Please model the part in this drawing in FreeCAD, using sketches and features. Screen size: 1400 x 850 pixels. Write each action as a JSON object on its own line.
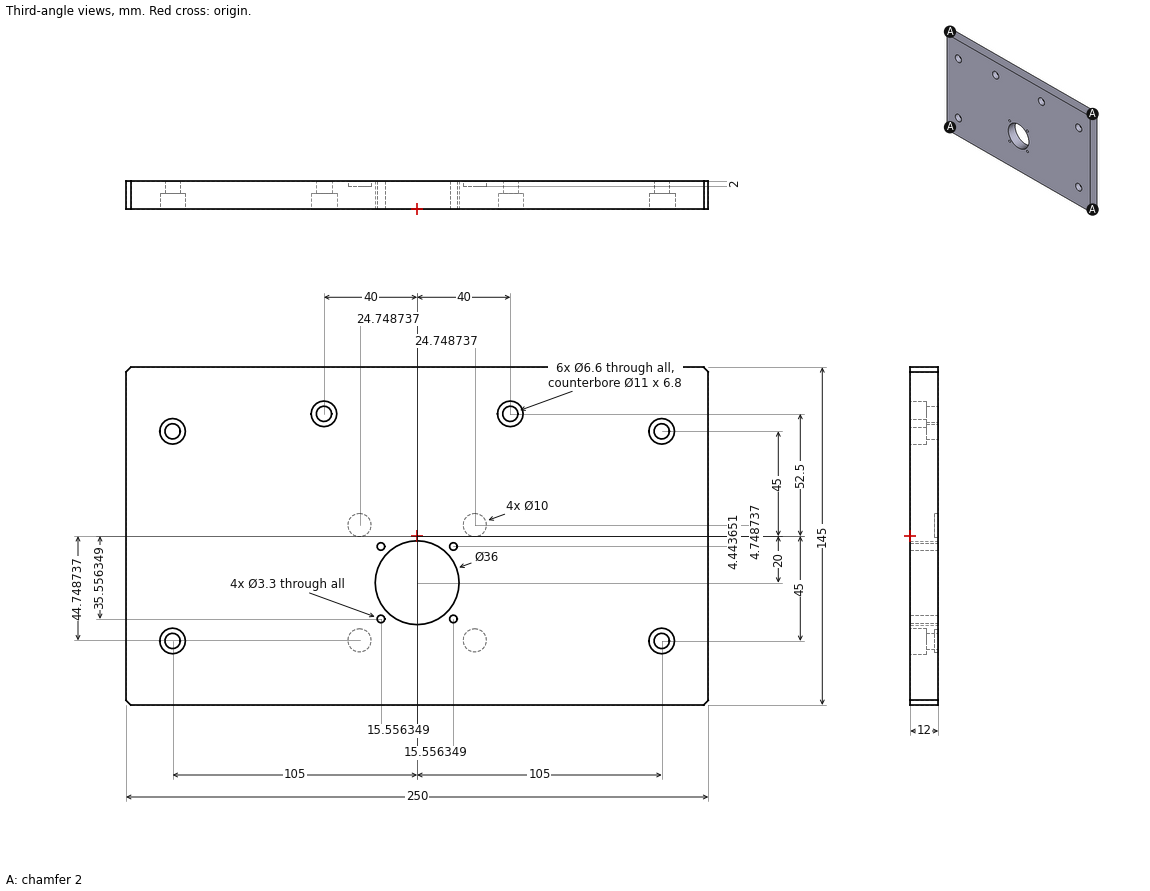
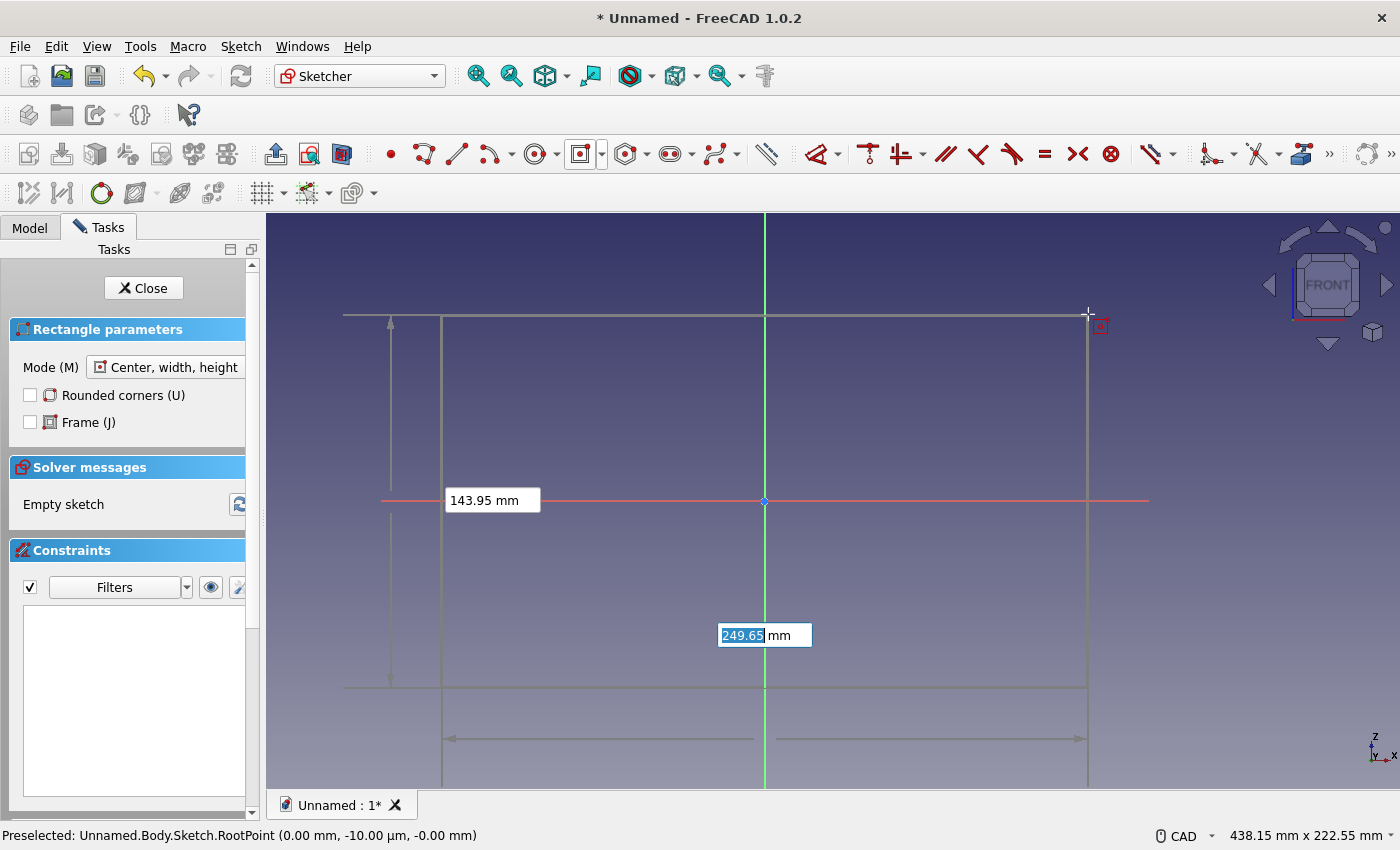
{"action": "type", "text": "250"}
{"action": "key", "text": "Tab"}
{"action": "type", "text": "145"}
{"action": "key", "text": "Return"}
{"action": "key", "text": "Escape"}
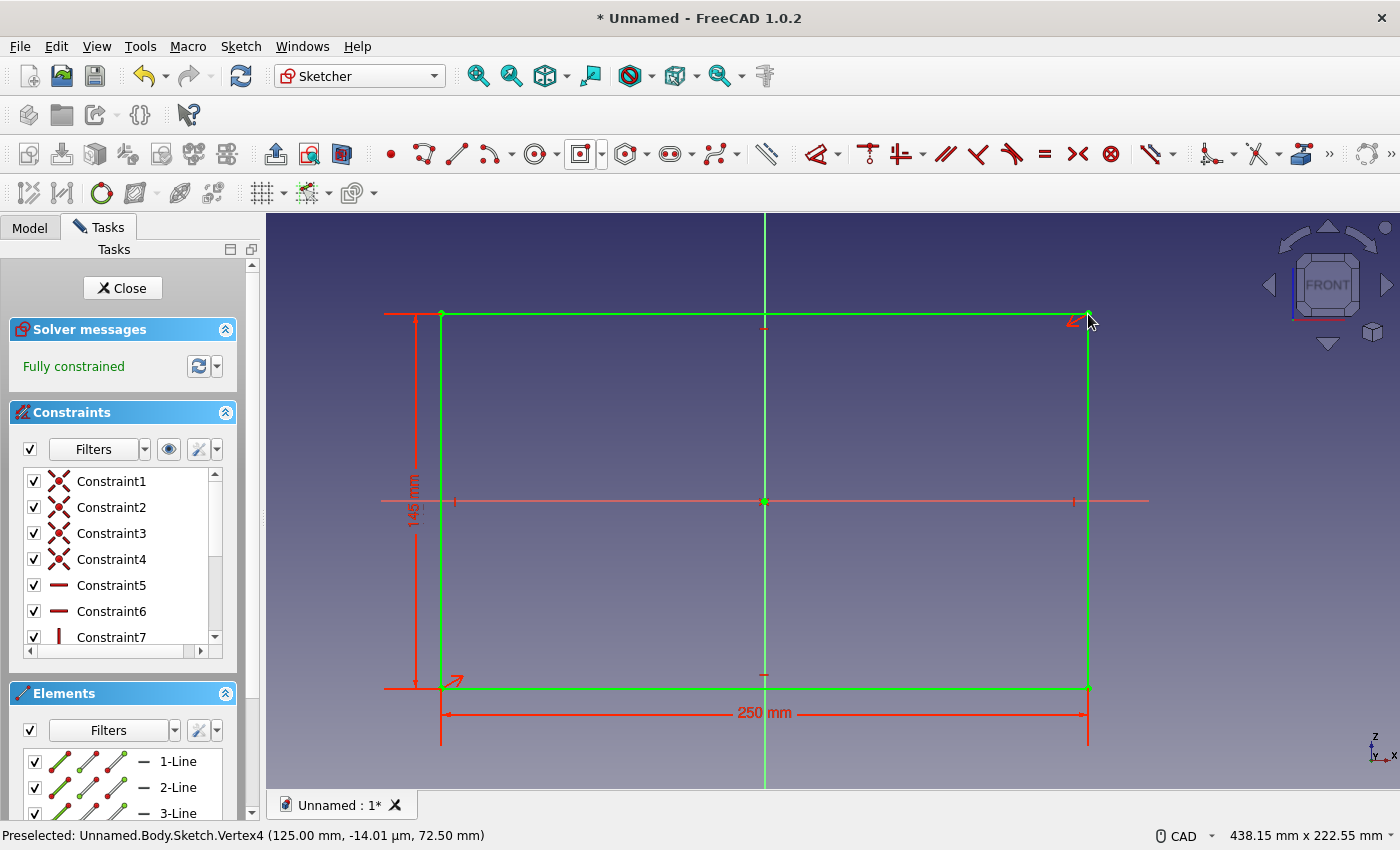
{"action": "left_click", "coordinate": [123, 288]}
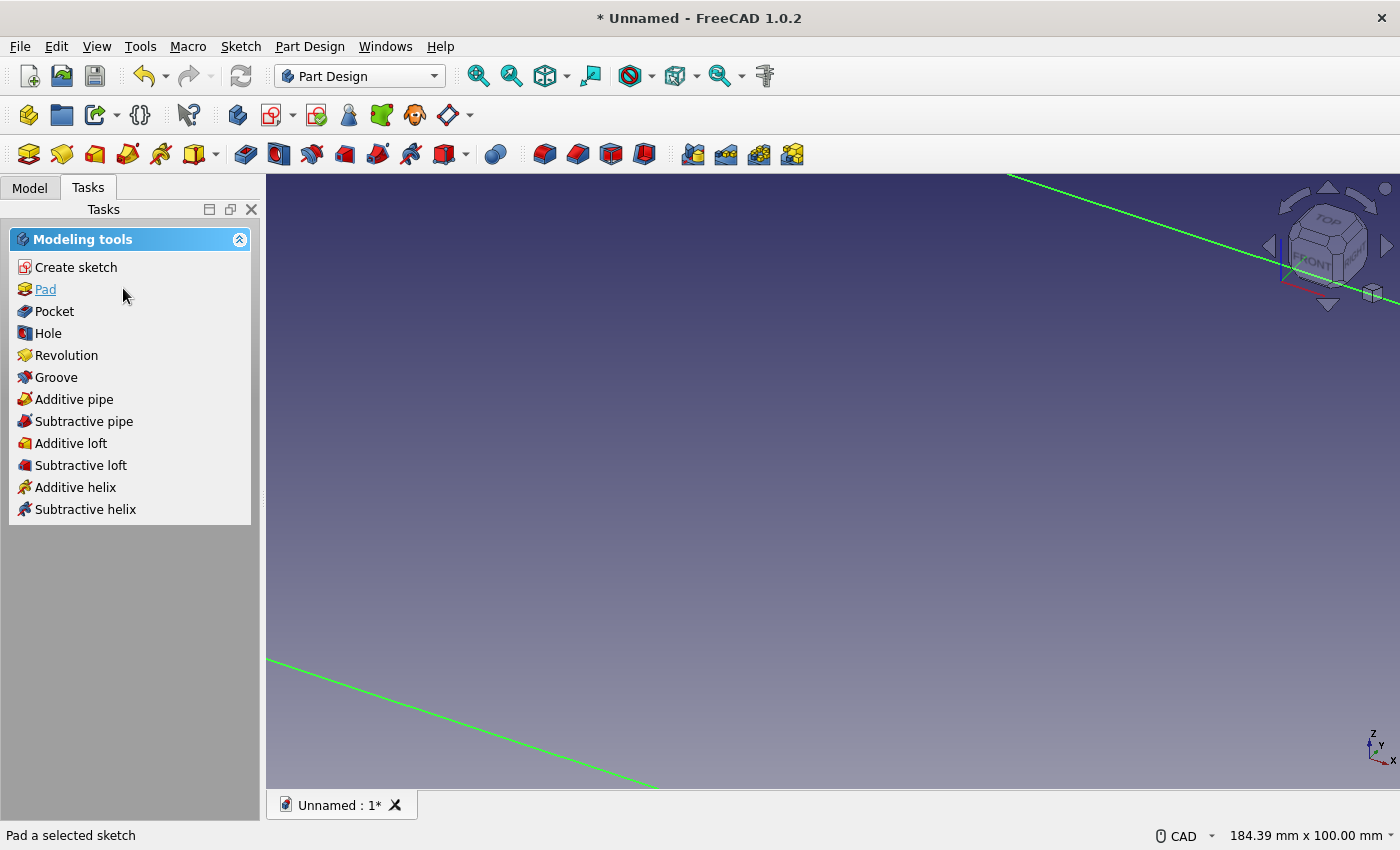
{"action": "left_click", "coordinate": [29, 154]}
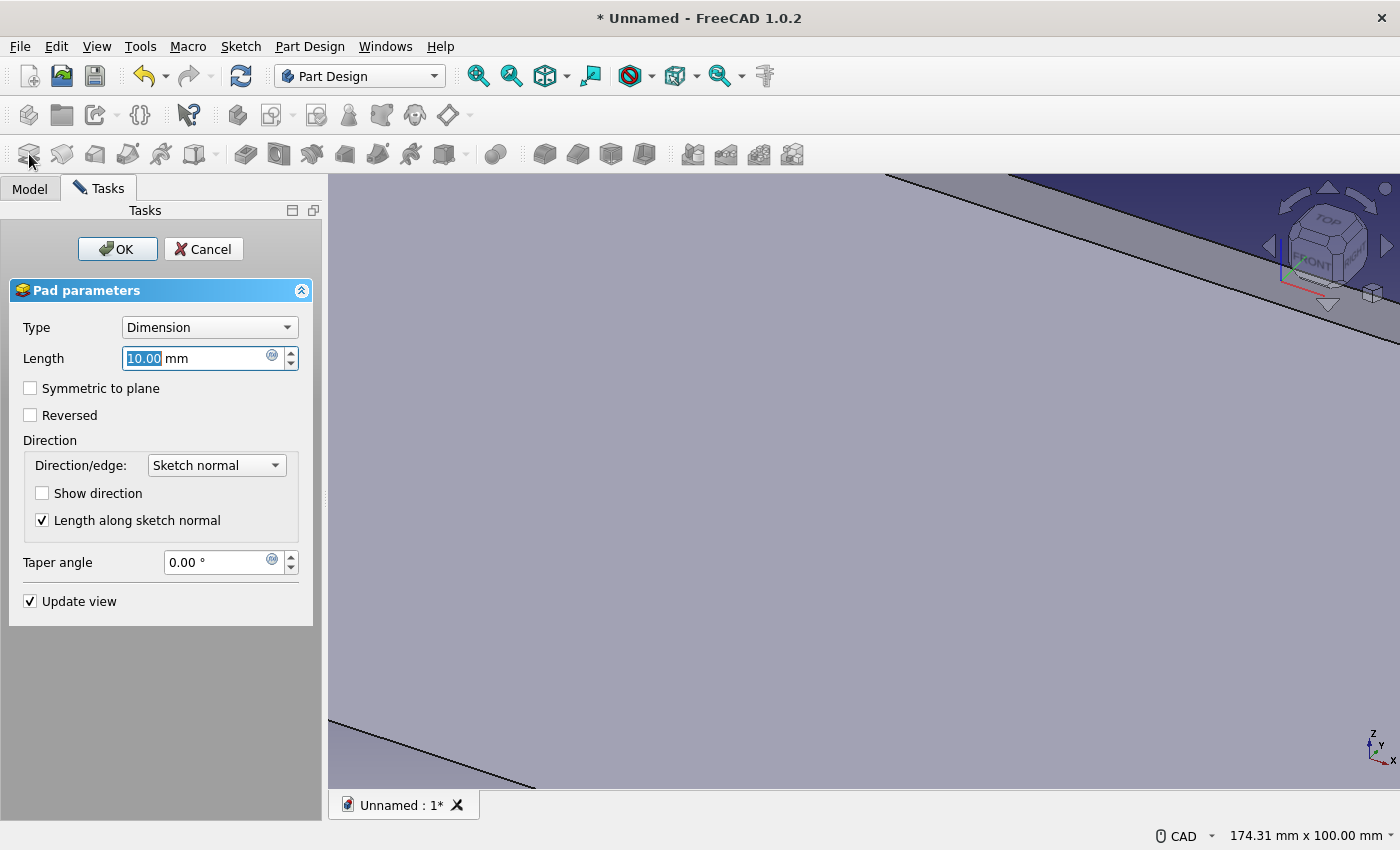
{"action": "type", "text": "12"}
{"action": "key", "text": "Tab"}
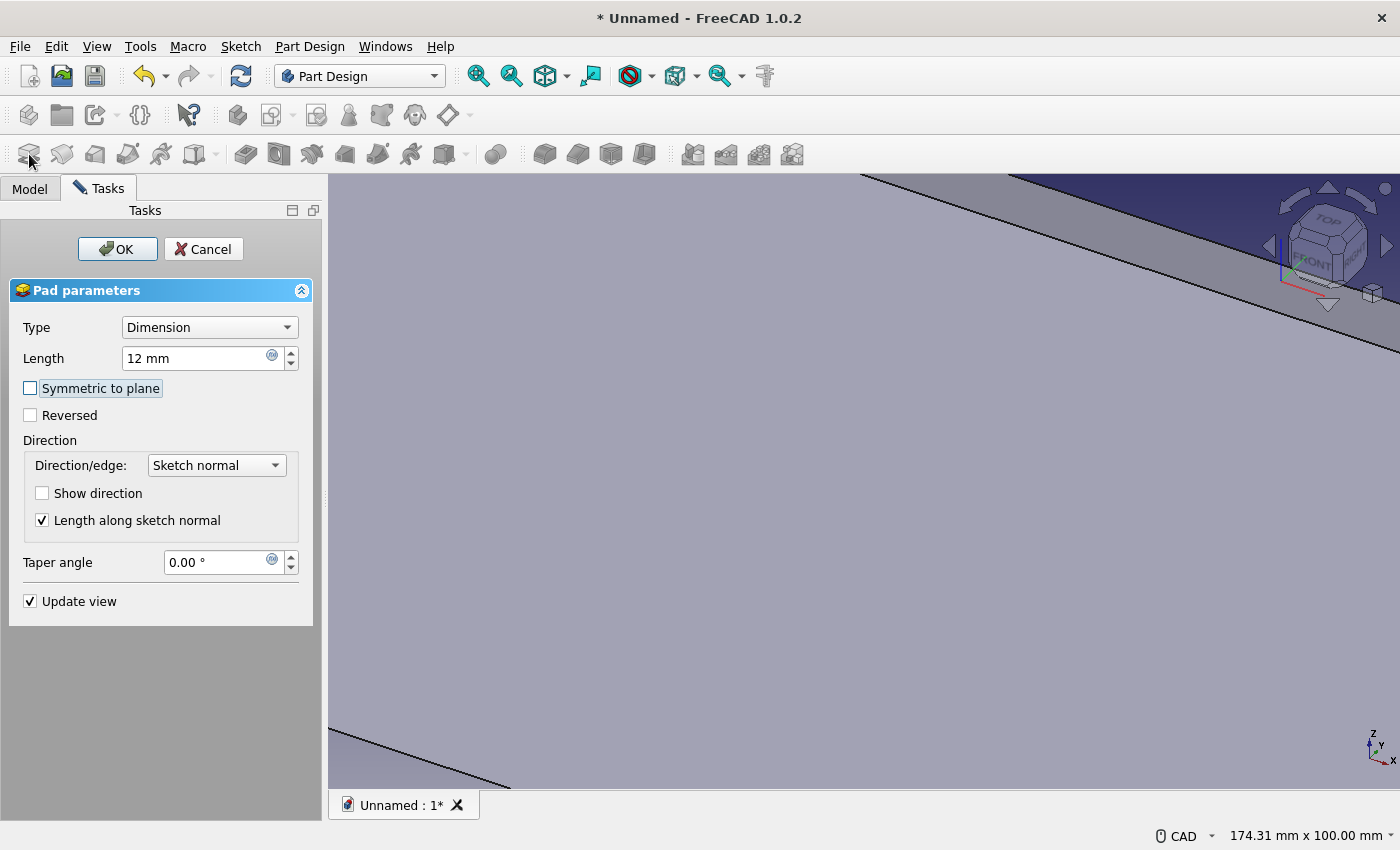
{"action": "left_click", "coordinate": [31, 415]}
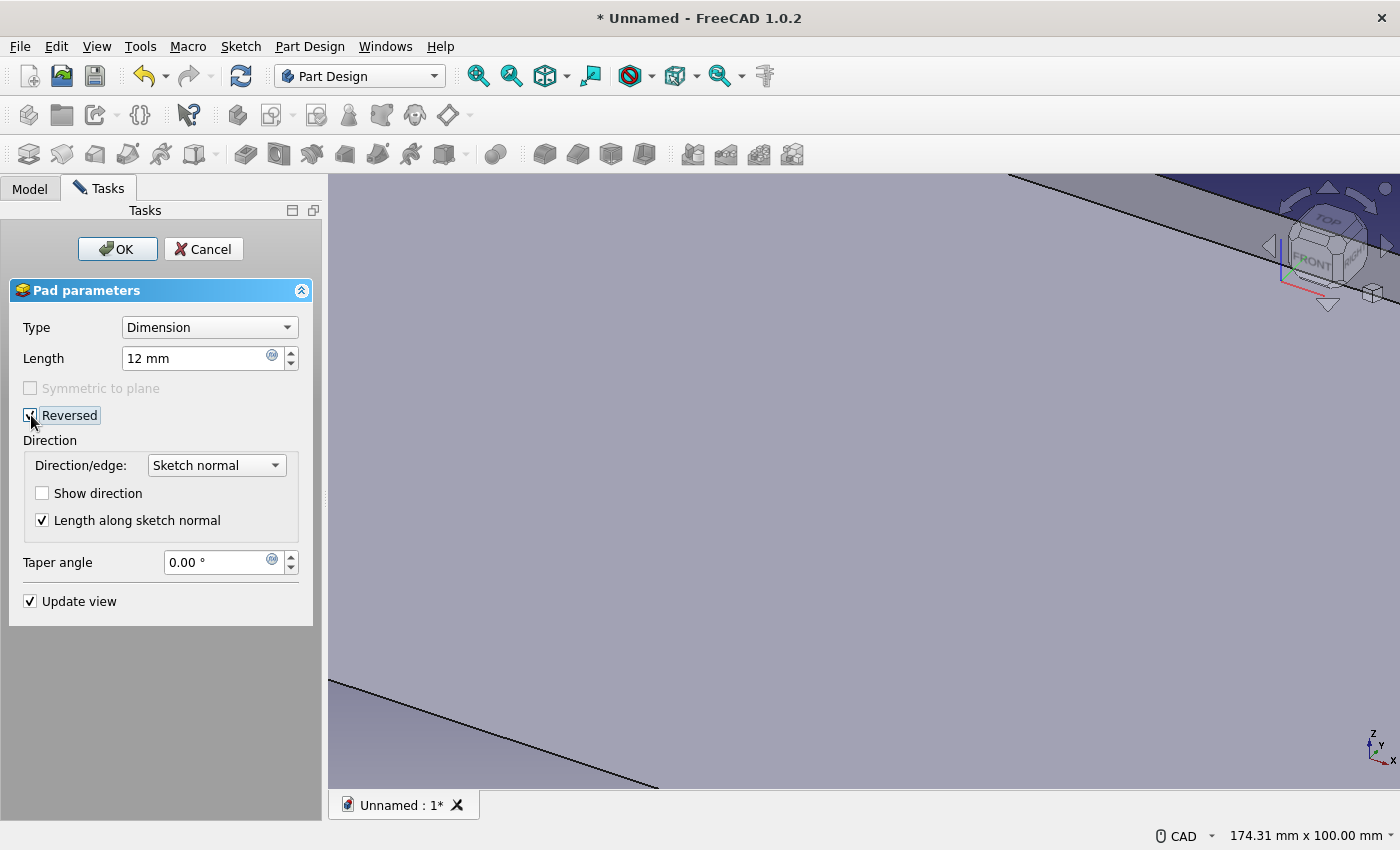
{"action": "left_click", "coordinate": [118, 249]}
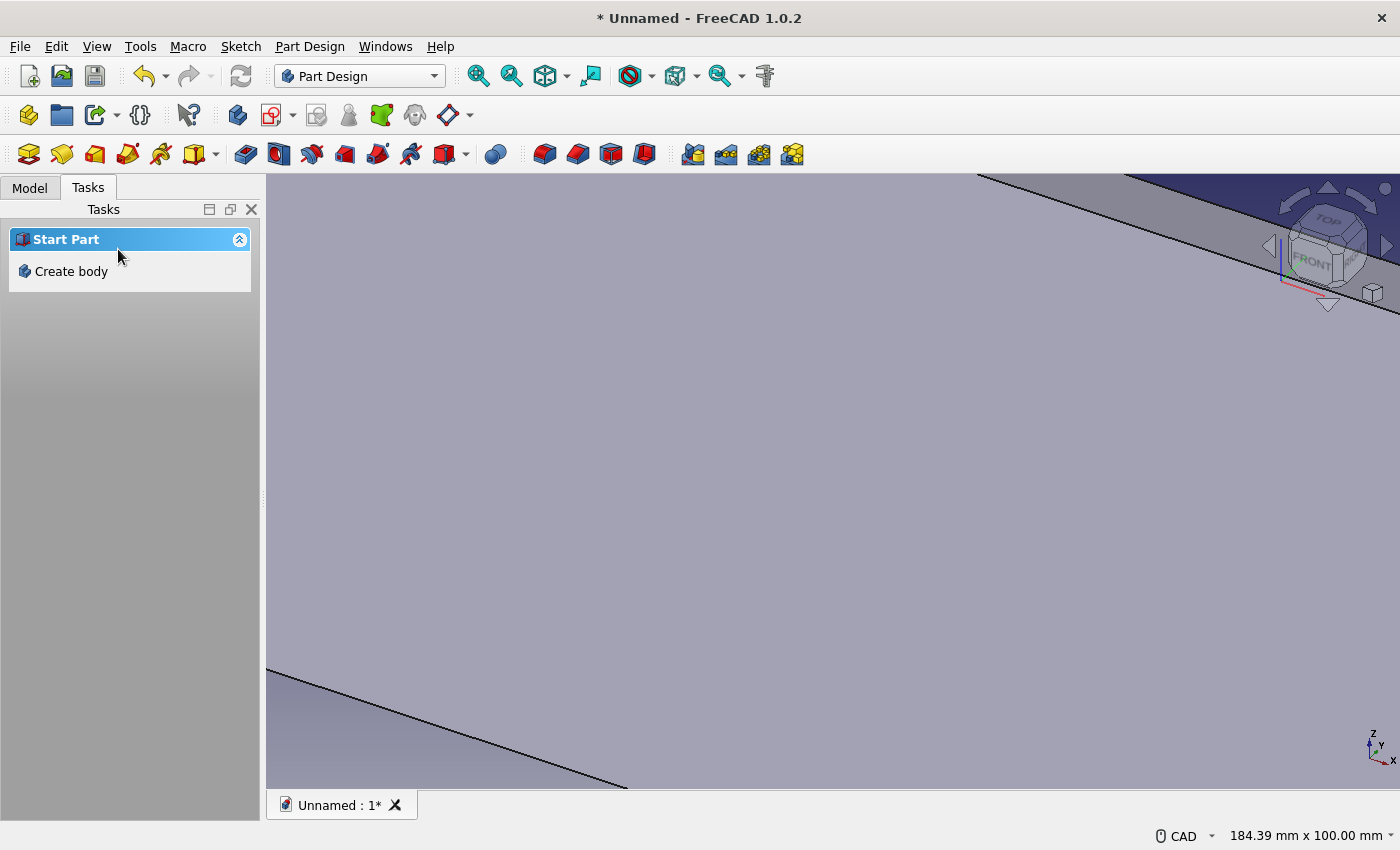
{"action": "left_click", "coordinate": [479, 76]}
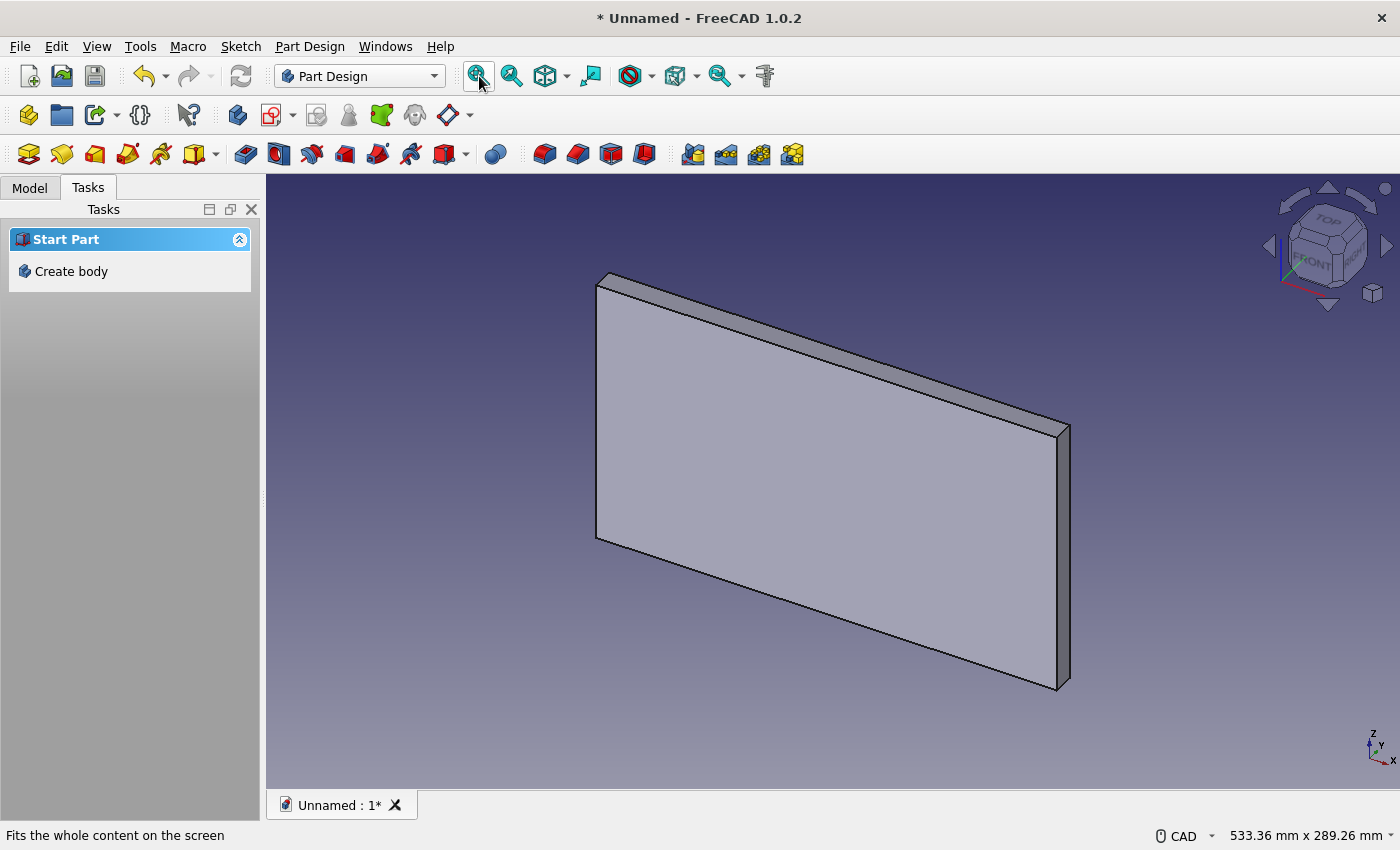
{"action": "left_click", "coordinate": [1063, 430]}